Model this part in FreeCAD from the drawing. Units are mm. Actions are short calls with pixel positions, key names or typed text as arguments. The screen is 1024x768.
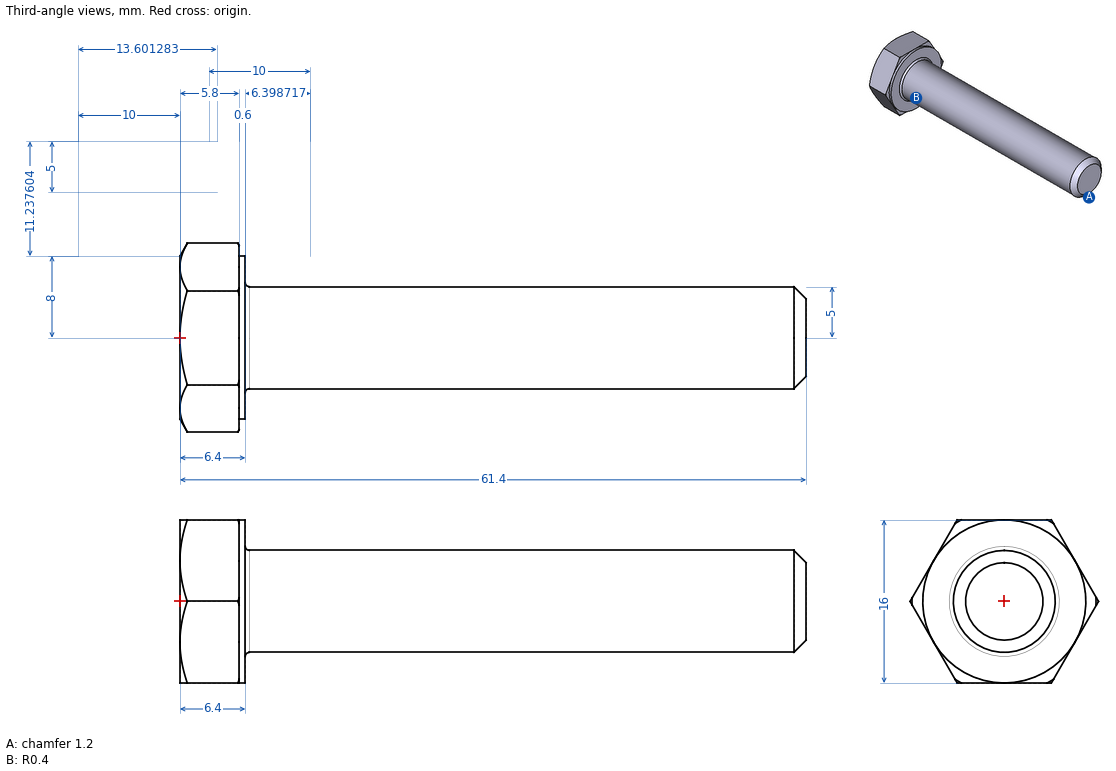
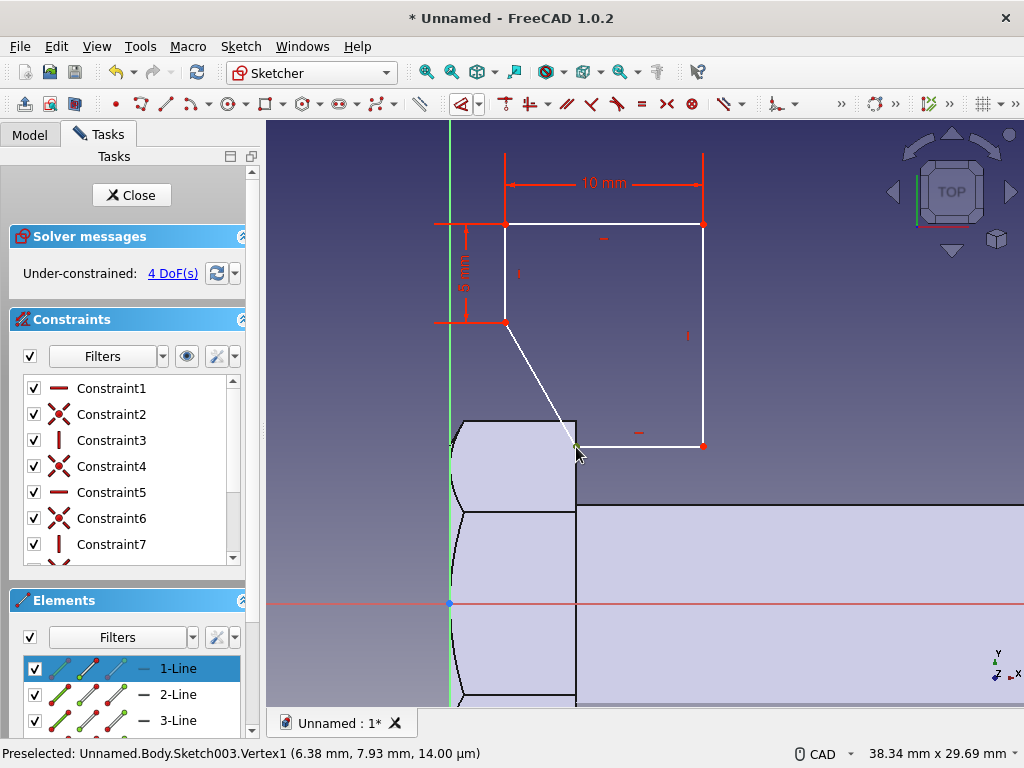
click(478, 104)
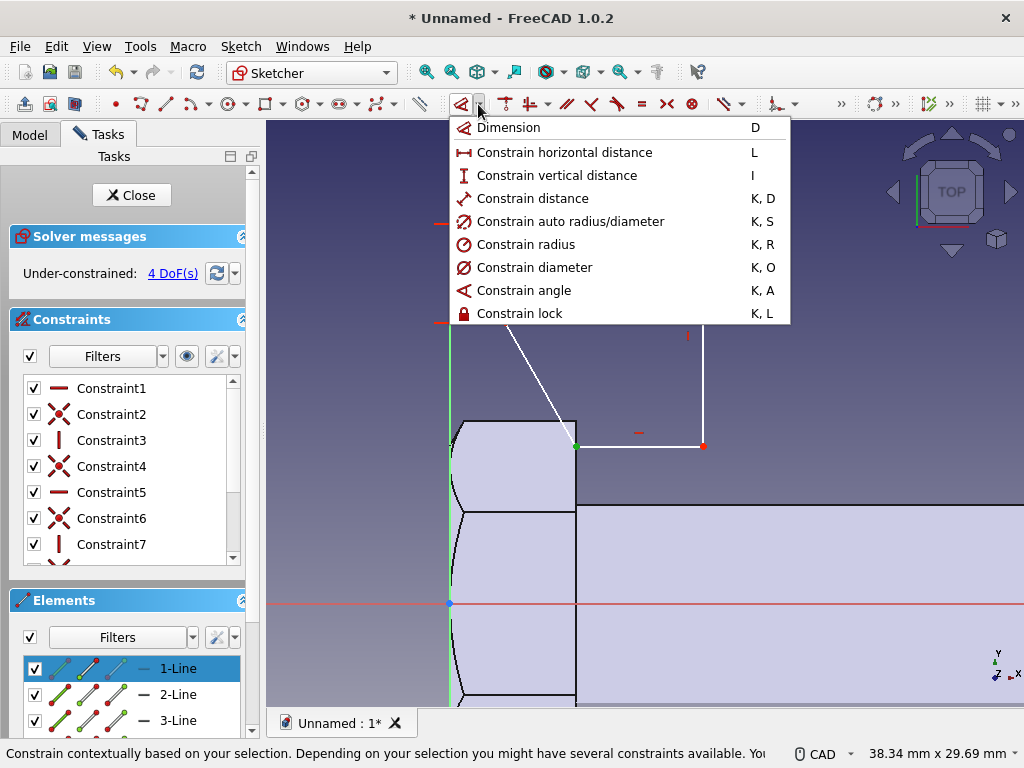
click(620, 176)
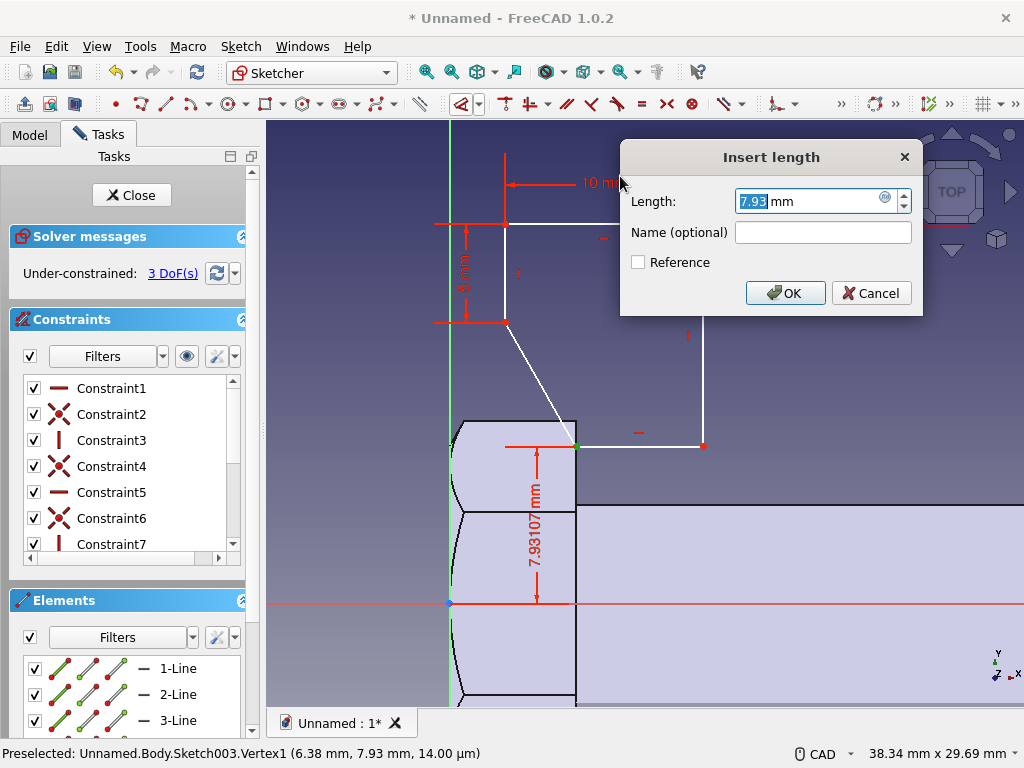
text(8)
key(Return)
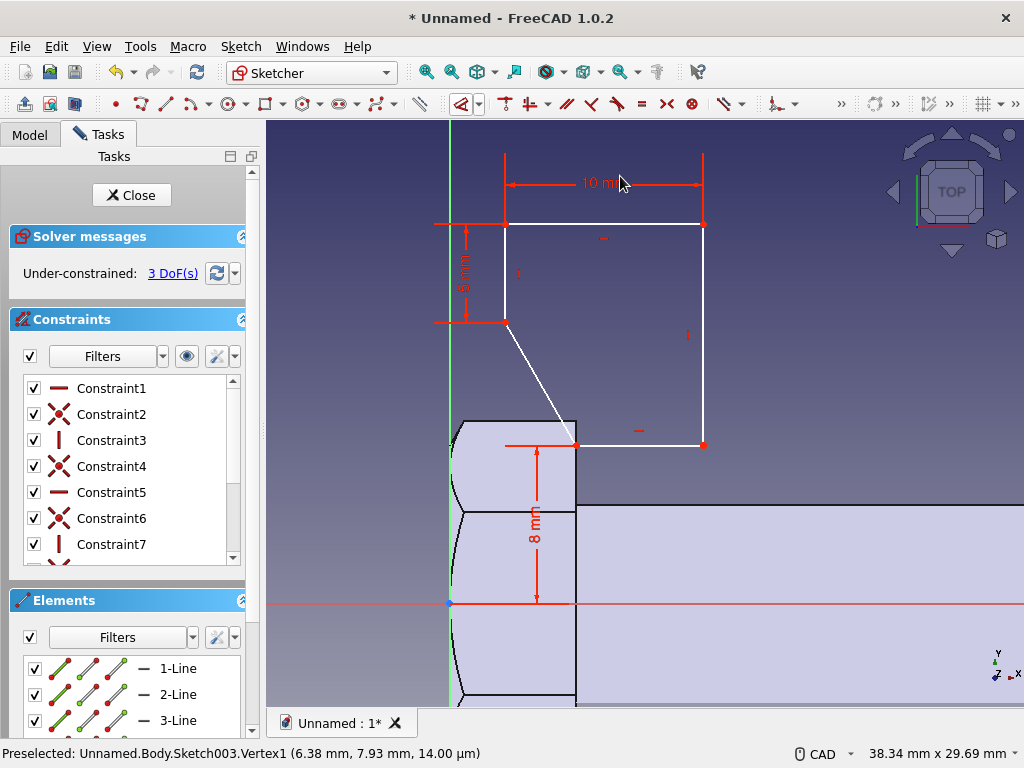
click(576, 446)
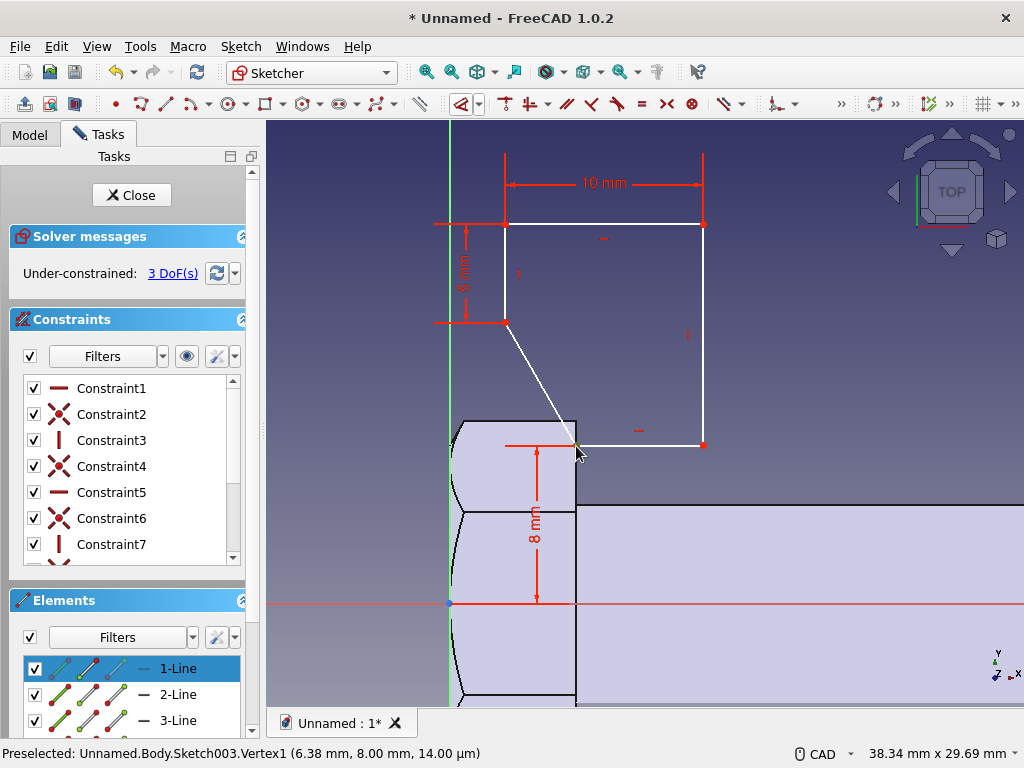
click(478, 104)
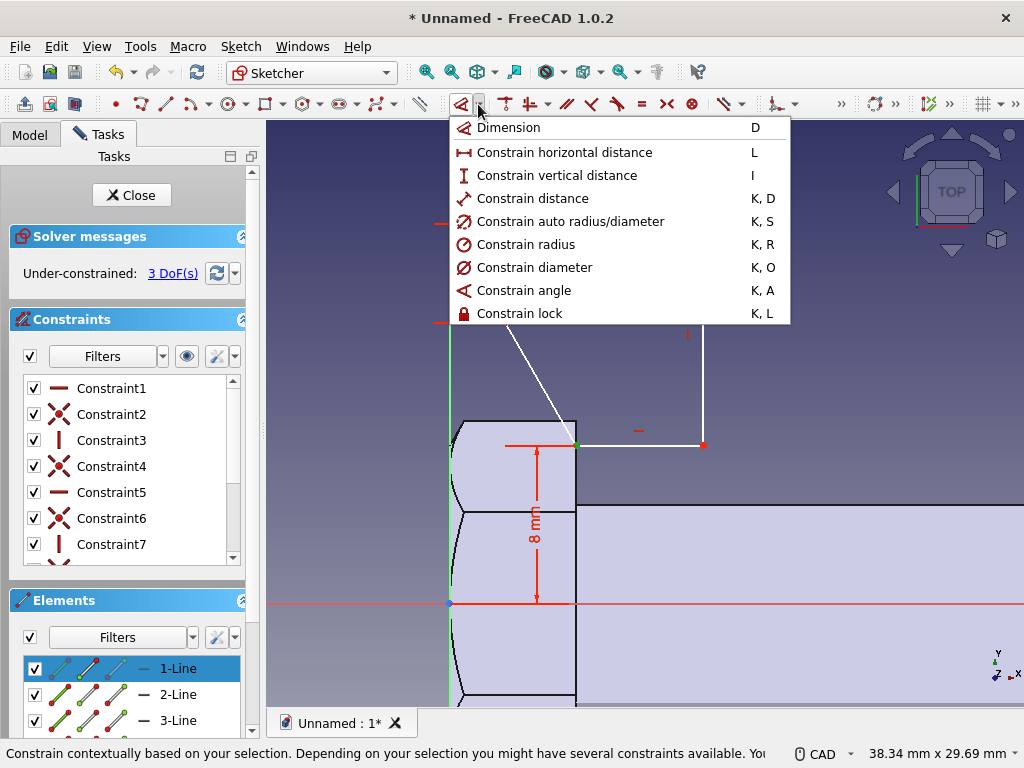
click(620, 152)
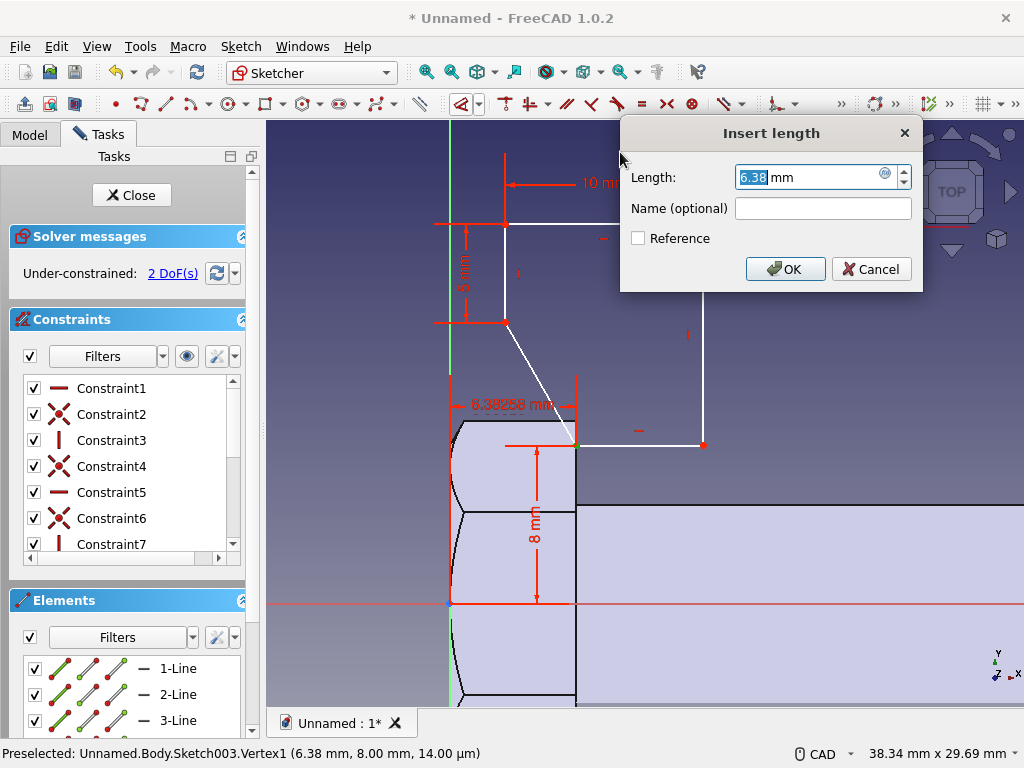
text(6.4)
key(Return)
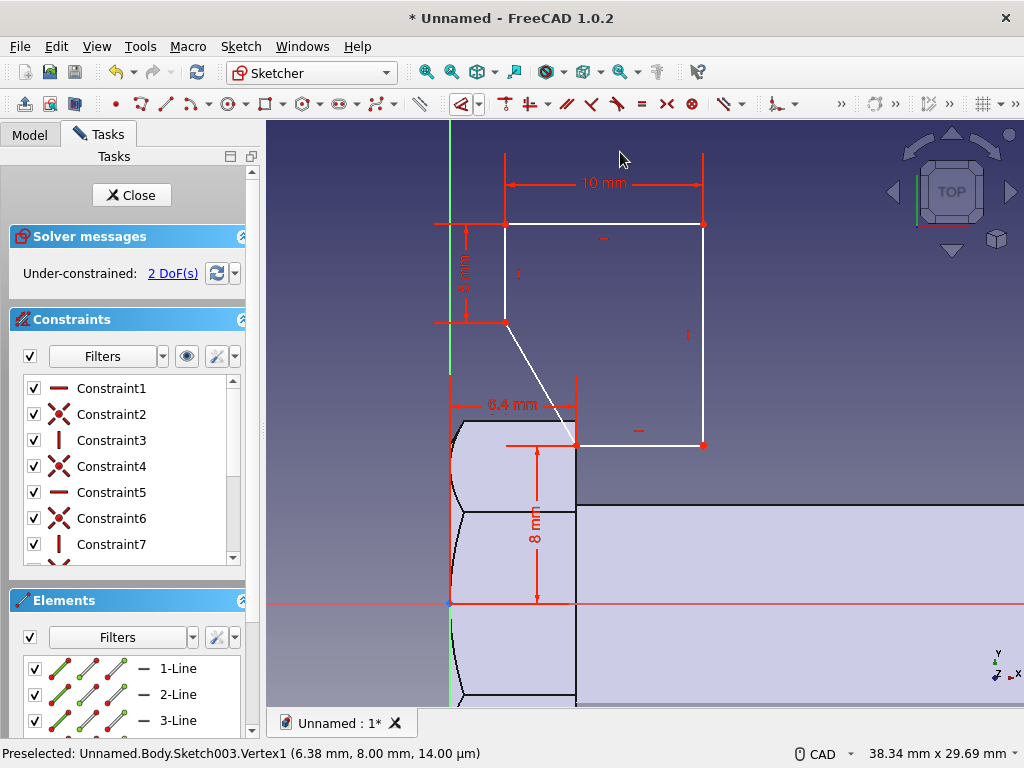
click(614, 446)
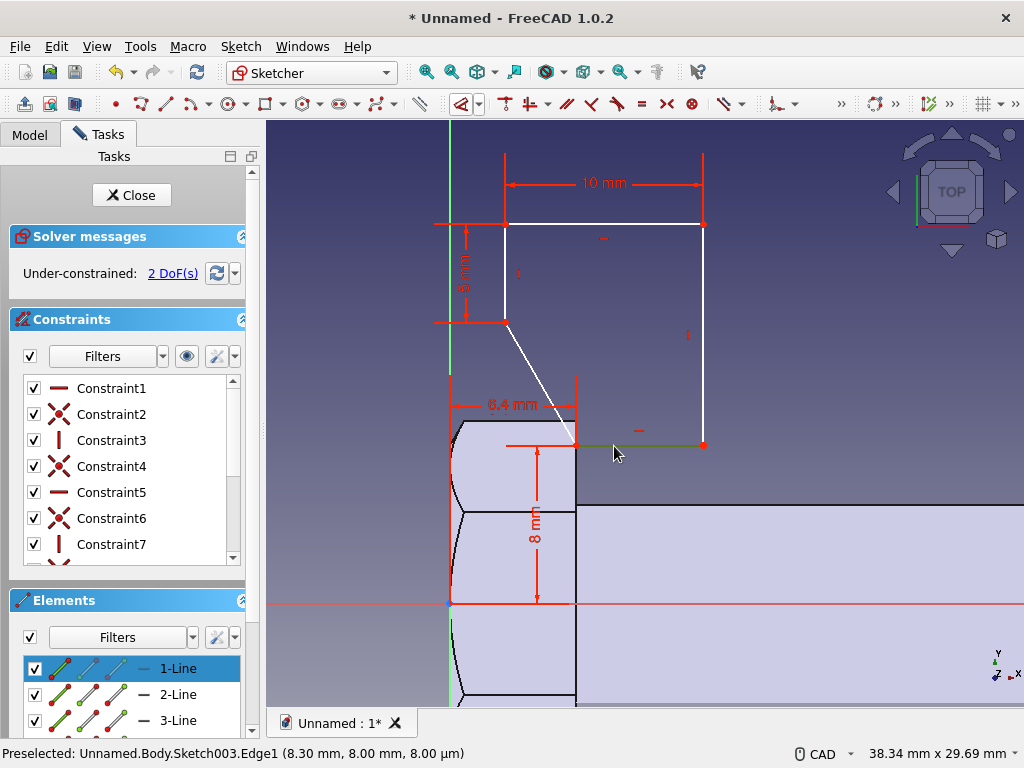
key(l)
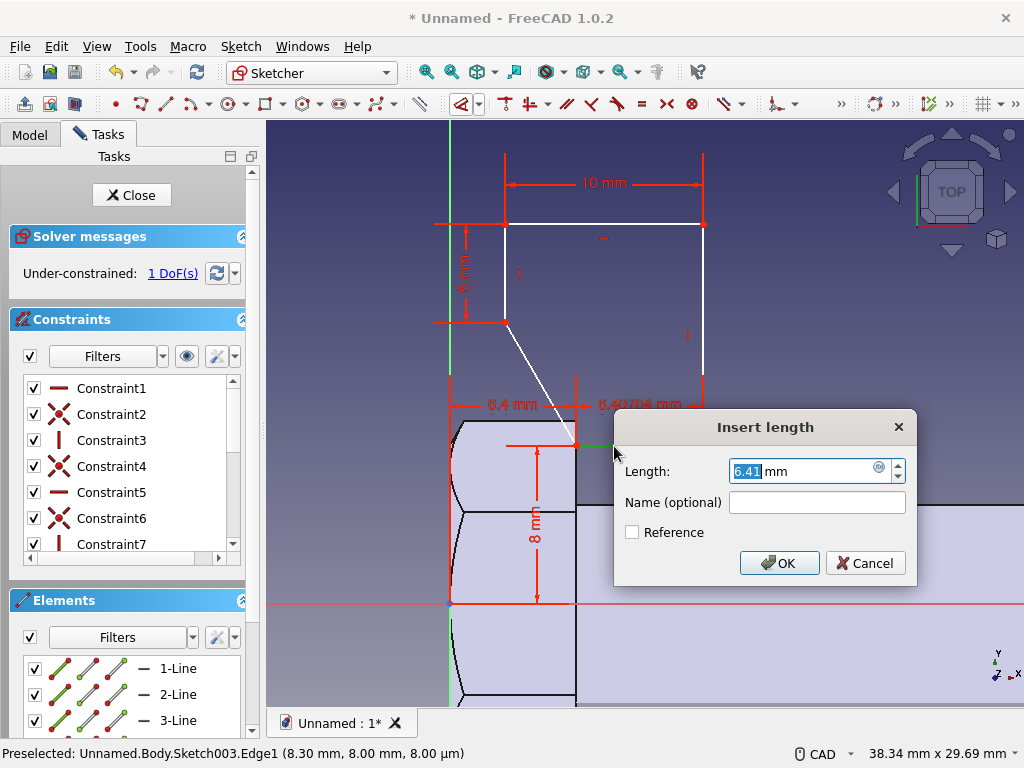
text(6.398717)
key(Return)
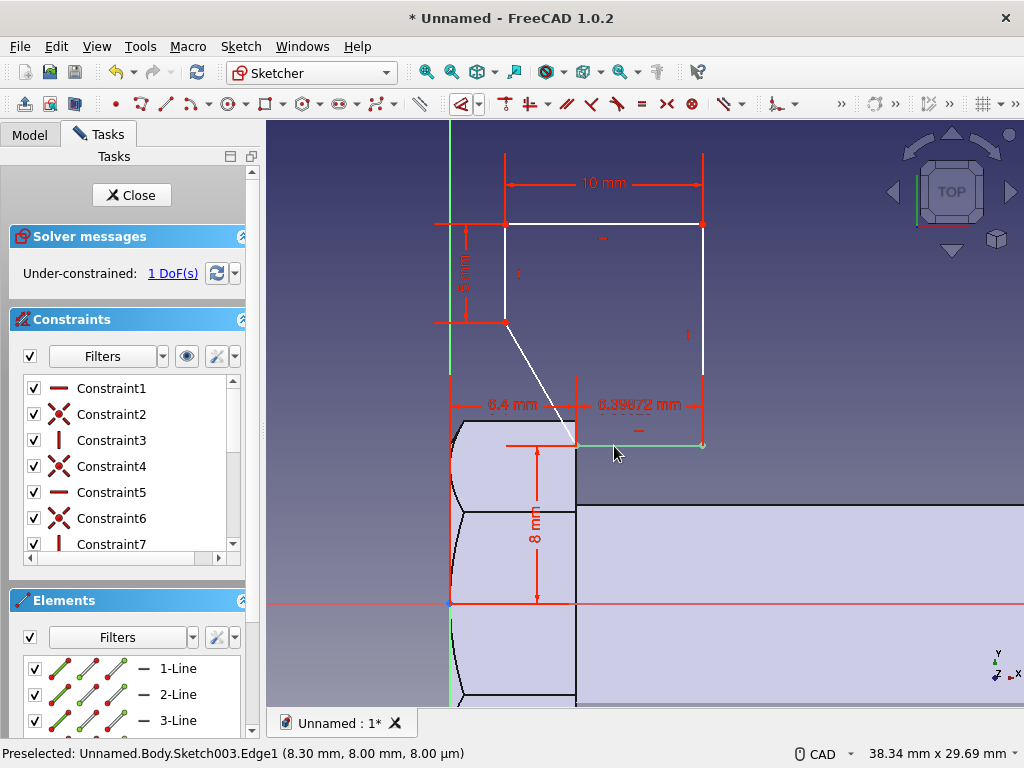
click(703, 379)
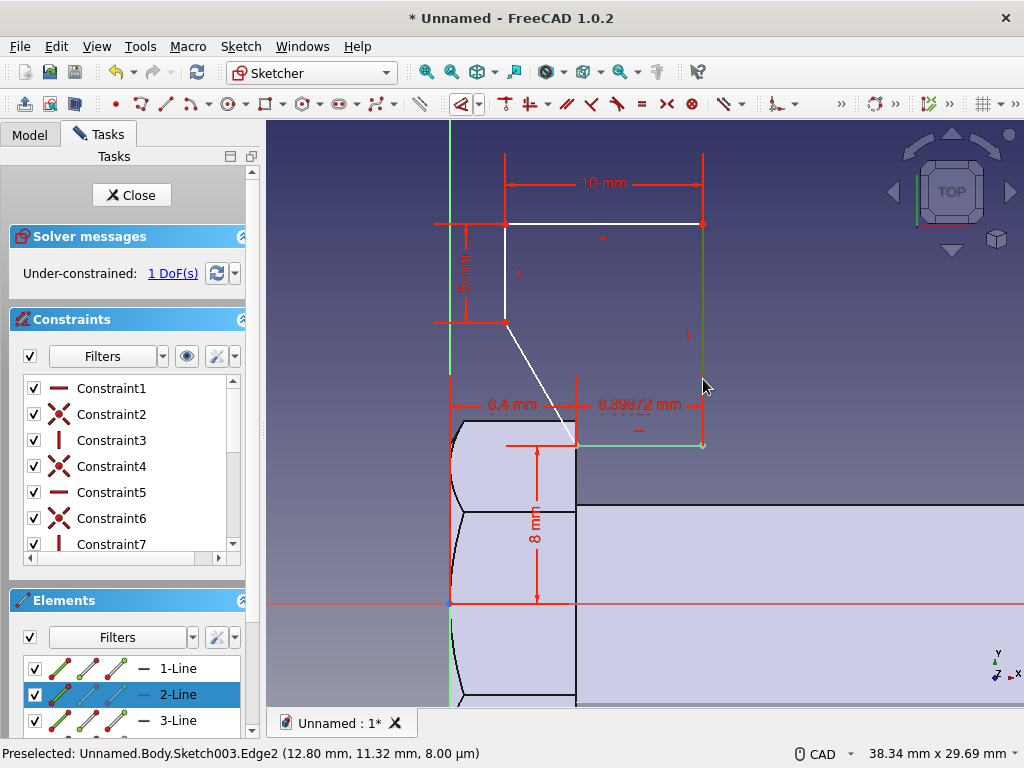
click(478, 104)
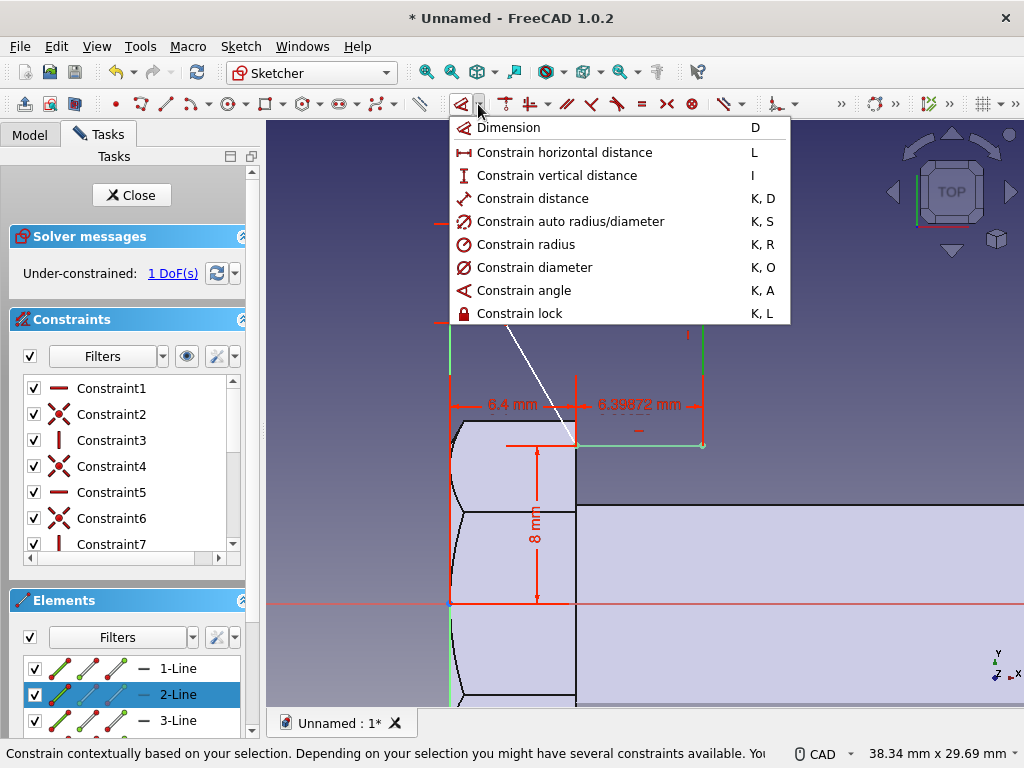
click(620, 176)